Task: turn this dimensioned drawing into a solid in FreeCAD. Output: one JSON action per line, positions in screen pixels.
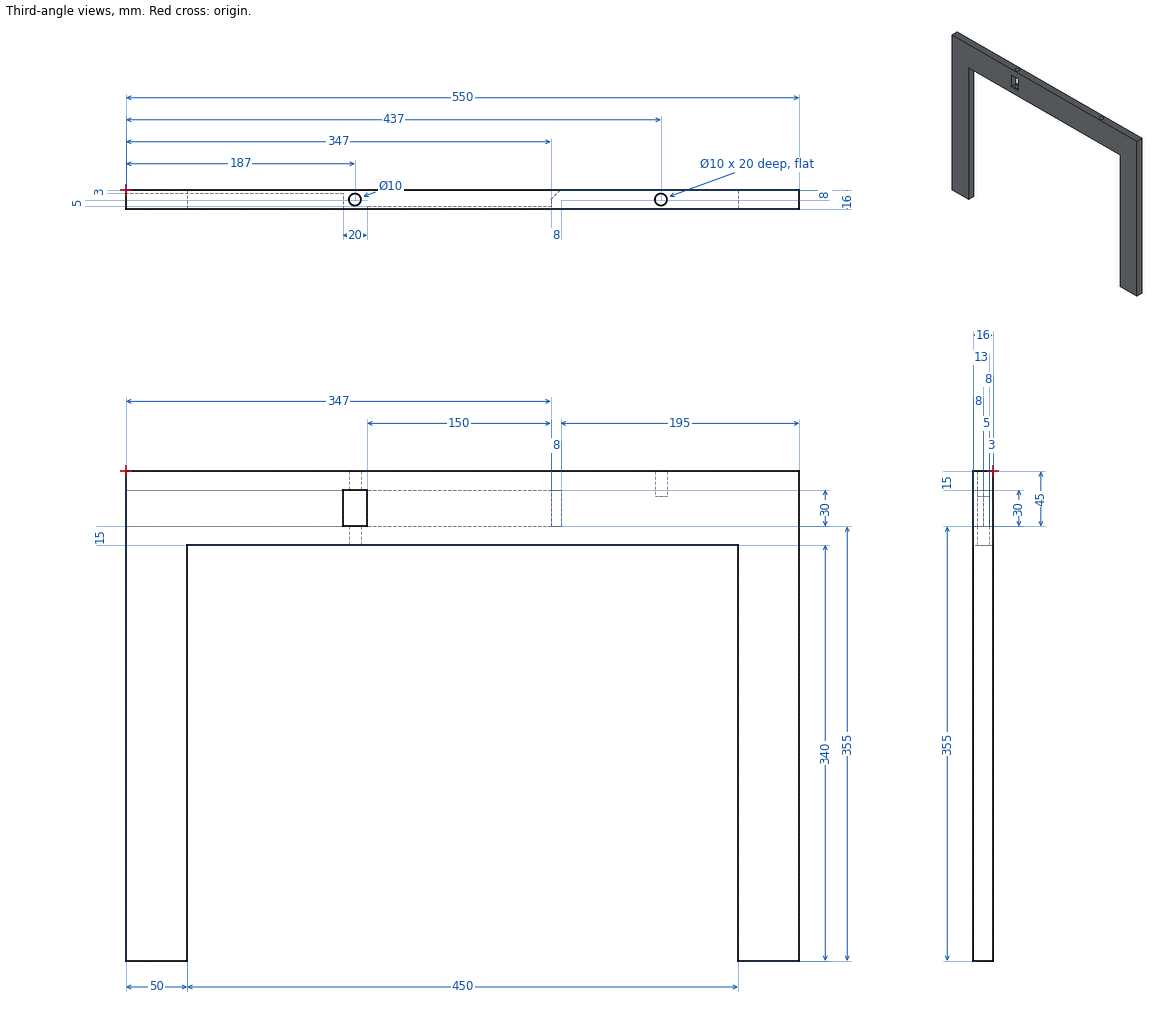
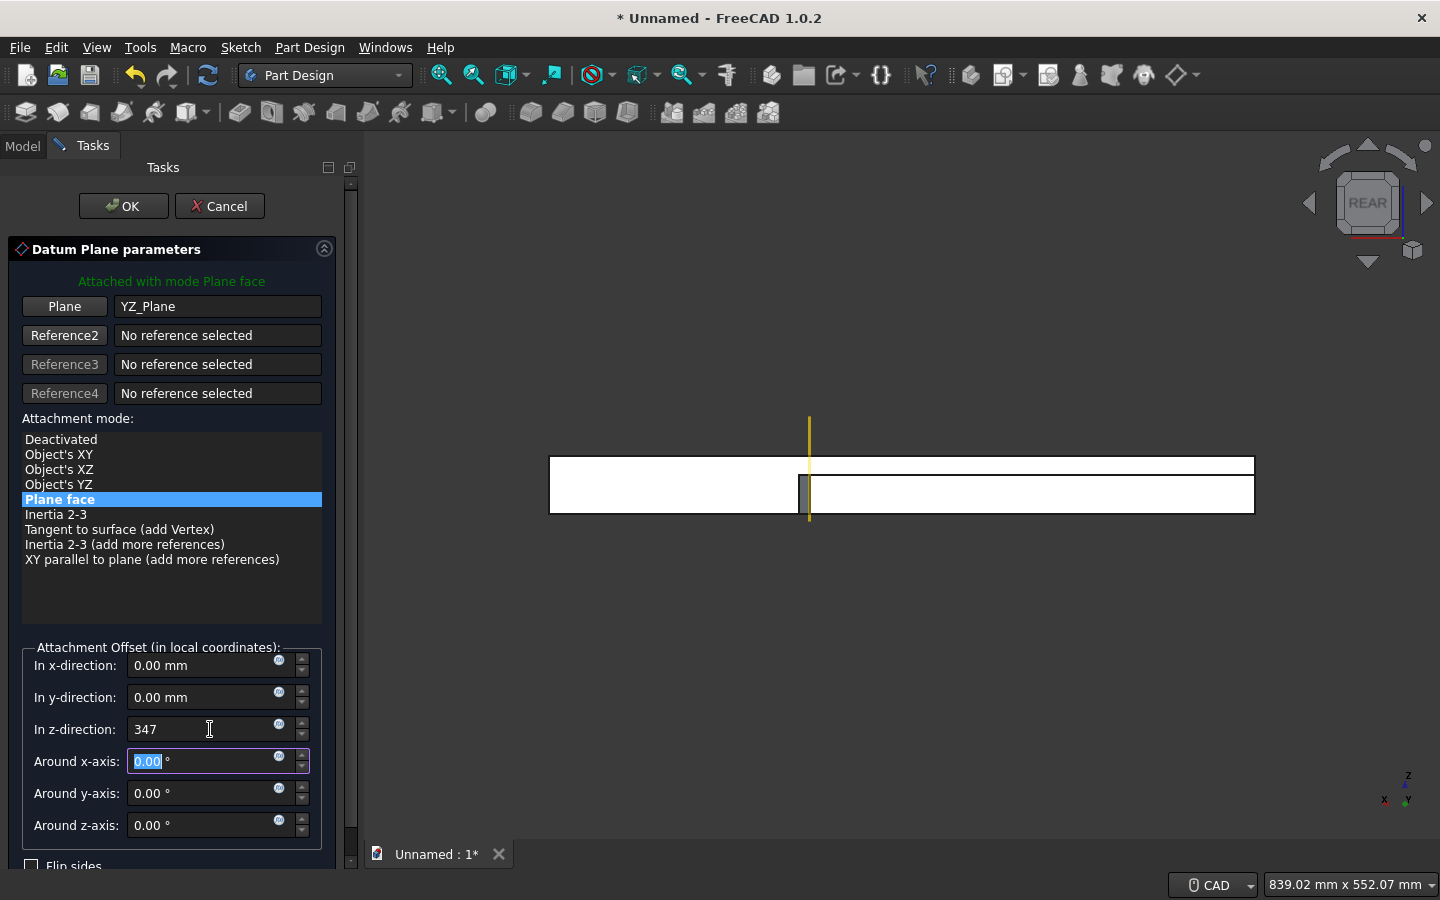
{"action": "left_click", "coordinate": [124, 206]}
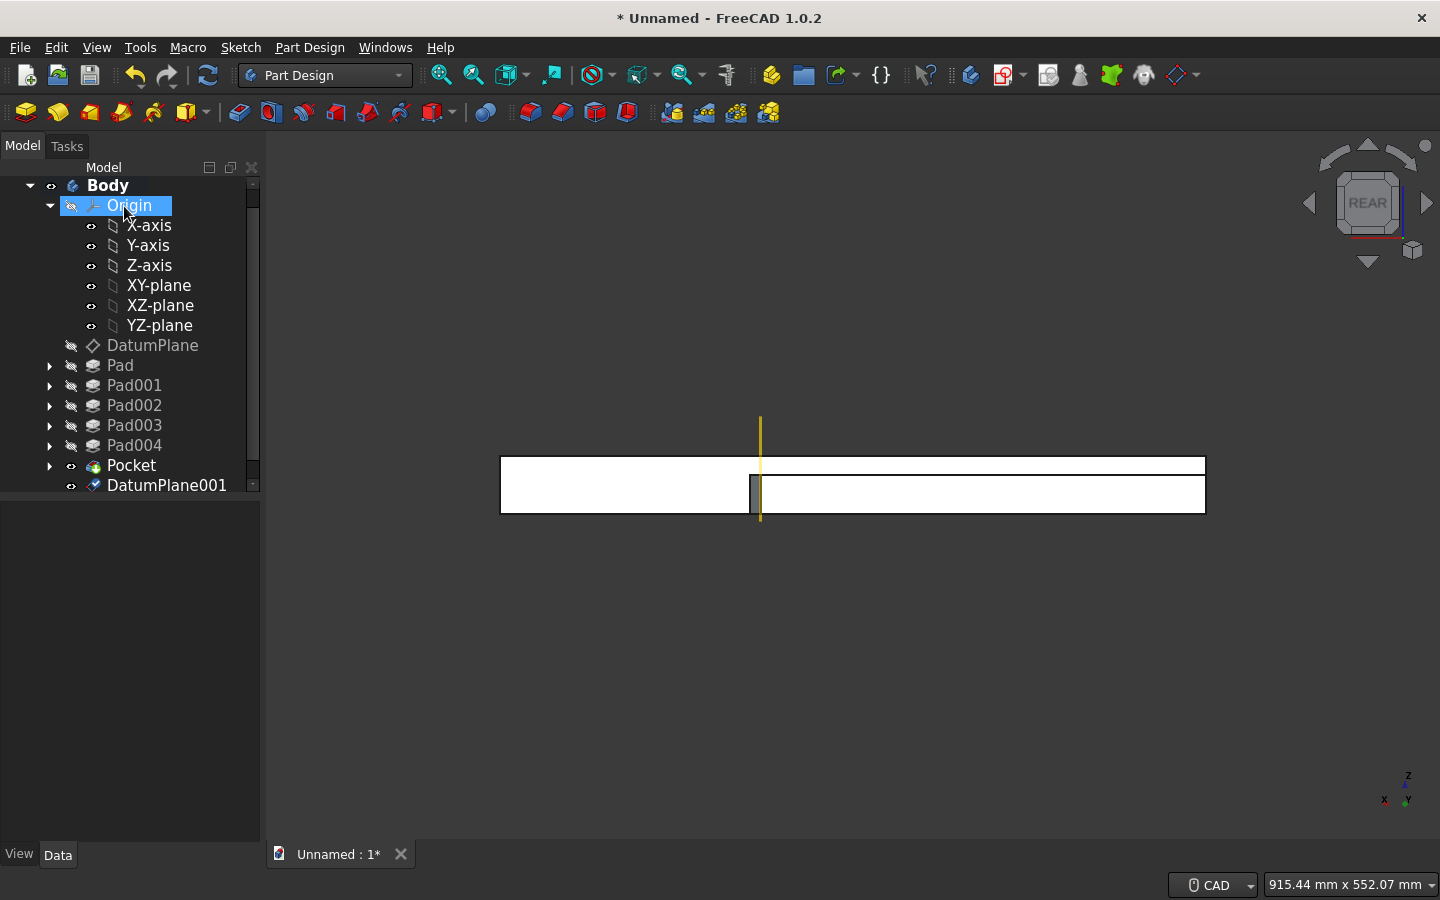
{"action": "left_click", "coordinate": [116, 486]}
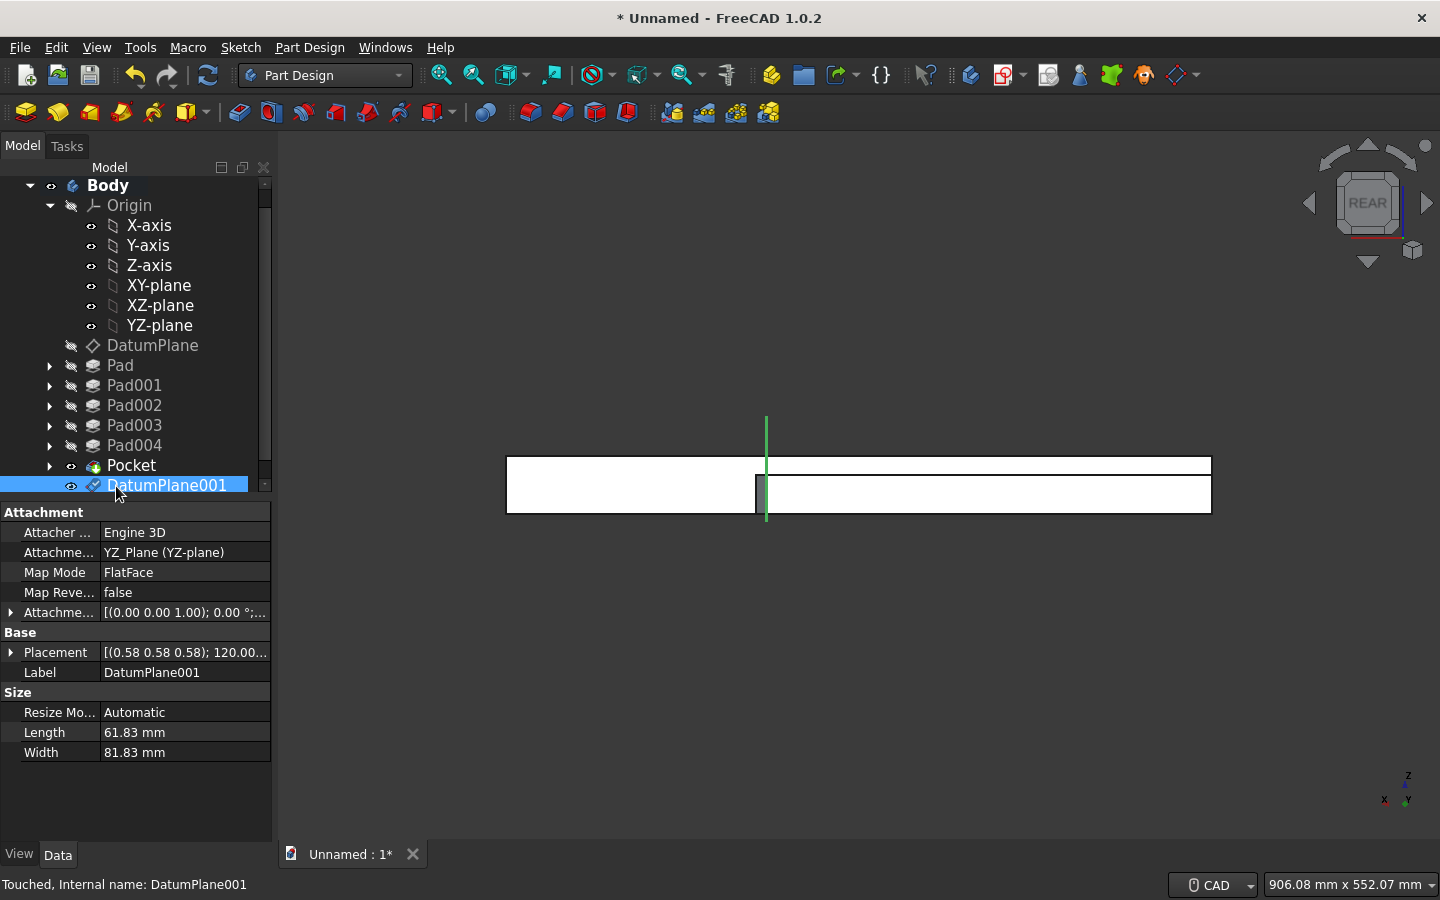
{"action": "left_click", "coordinate": [1004, 76]}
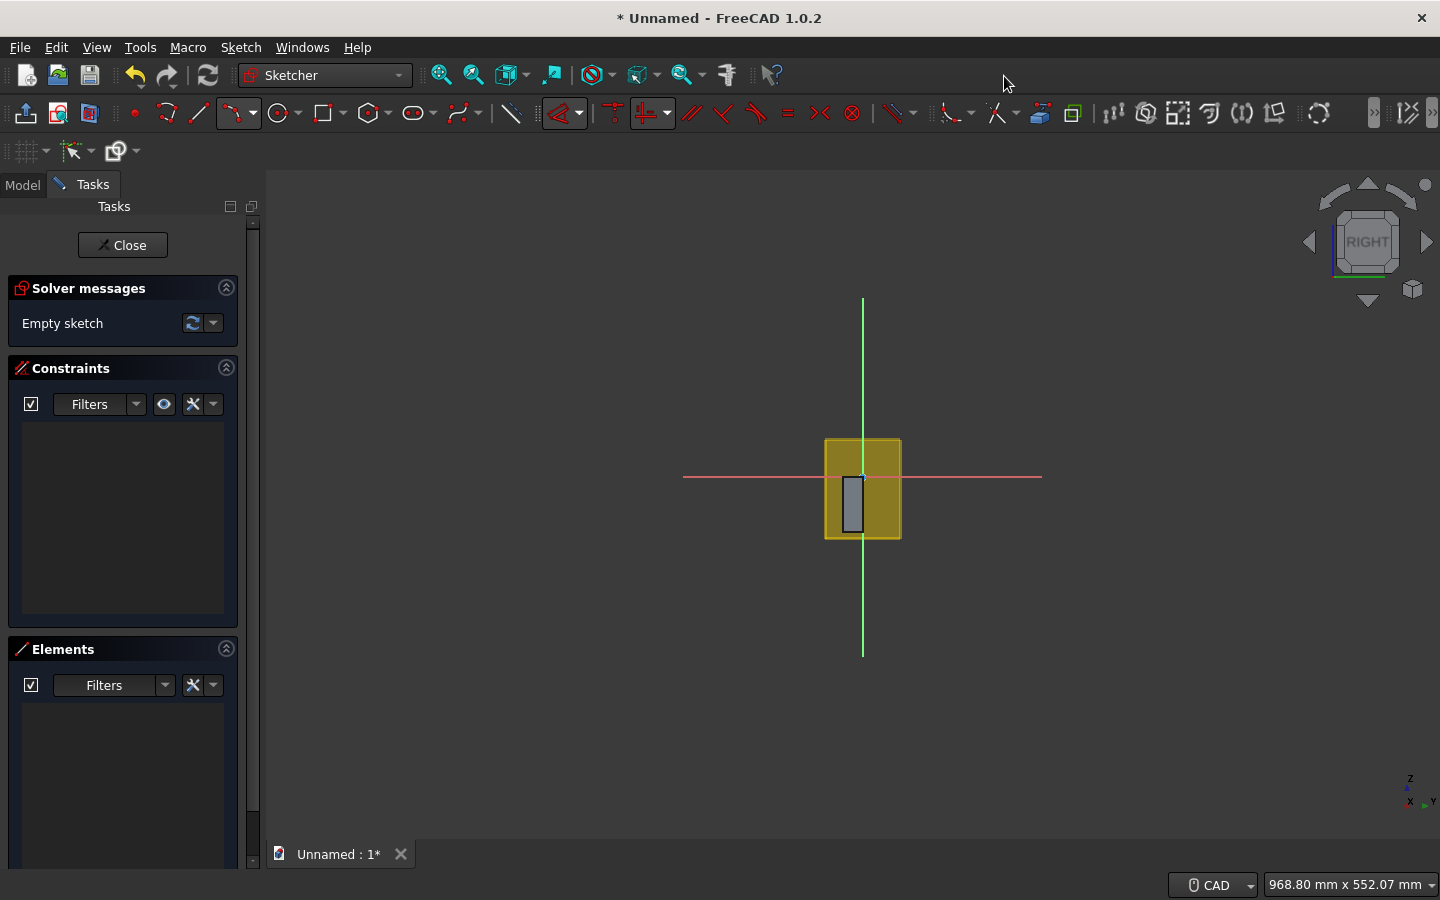
{"action": "left_click", "coordinate": [90, 114]}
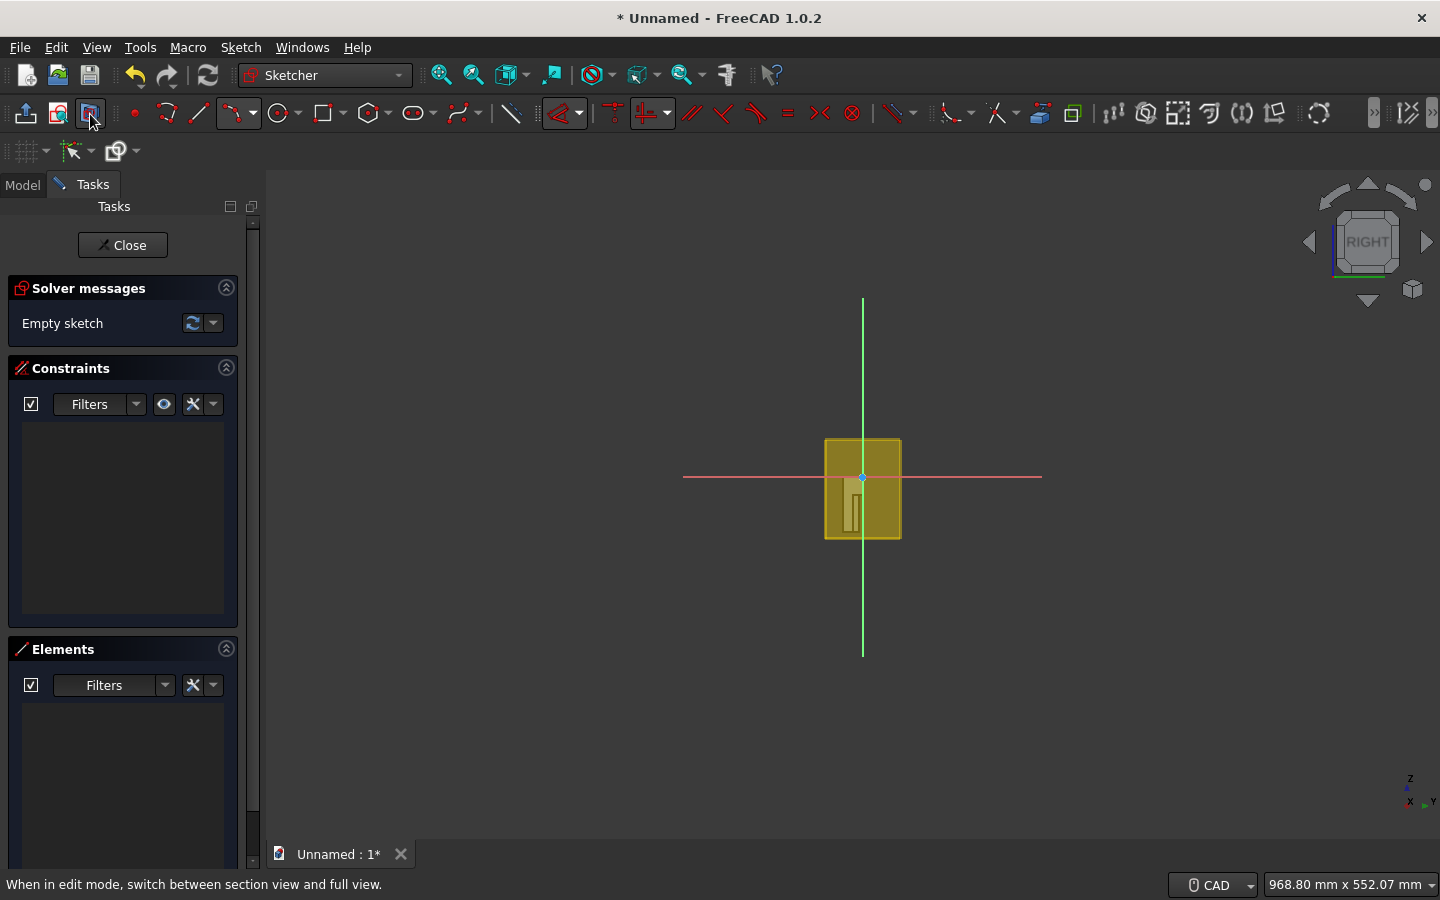
{"action": "scroll", "coordinate": [869, 505], "scroll_direction": "up", "scroll_amount": 10}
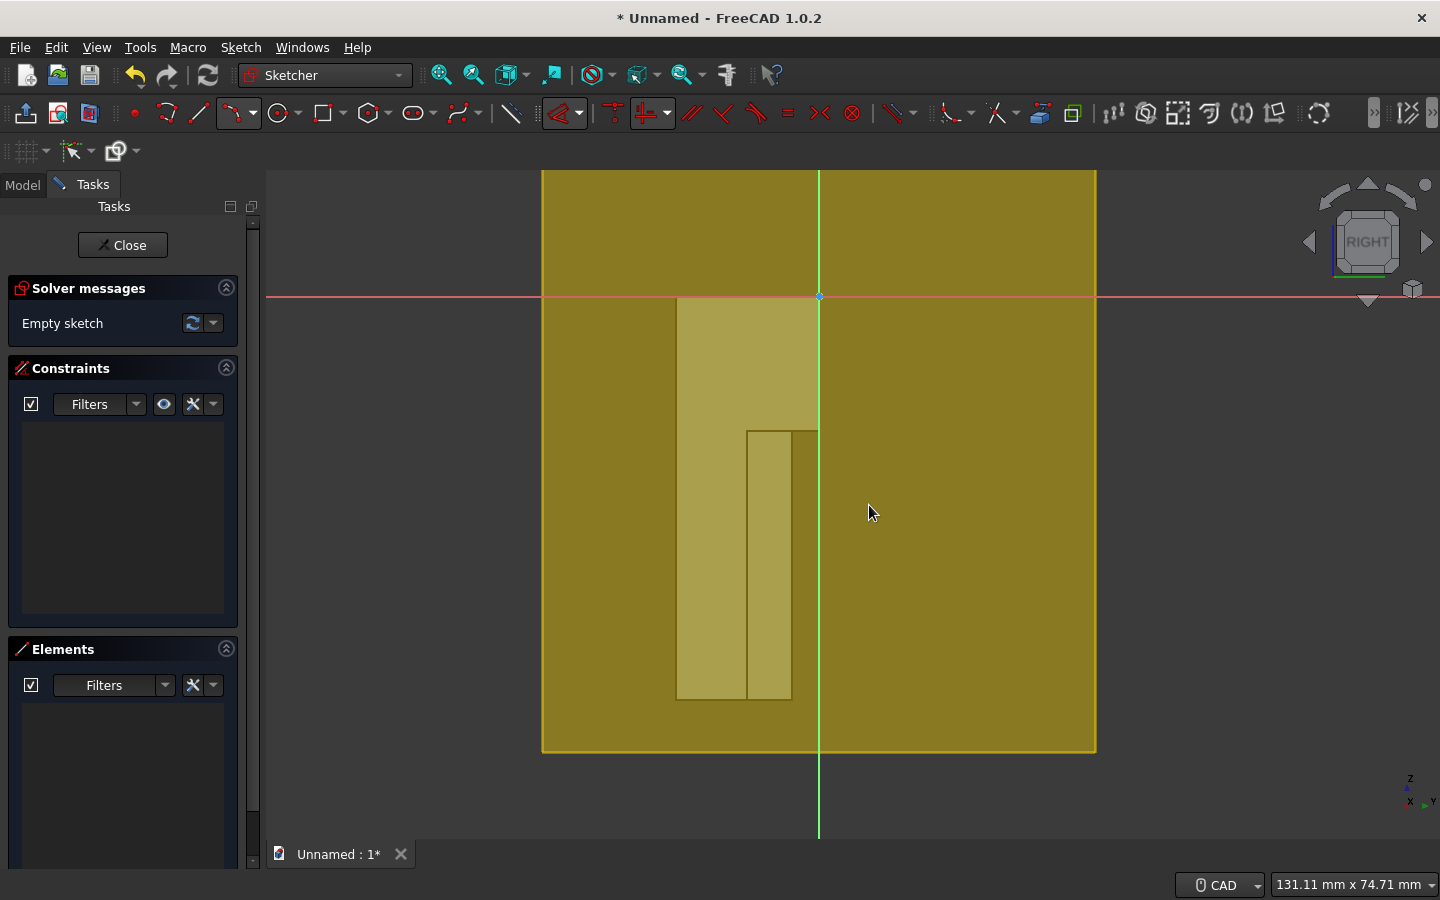
{"action": "left_click", "coordinate": [324, 114]}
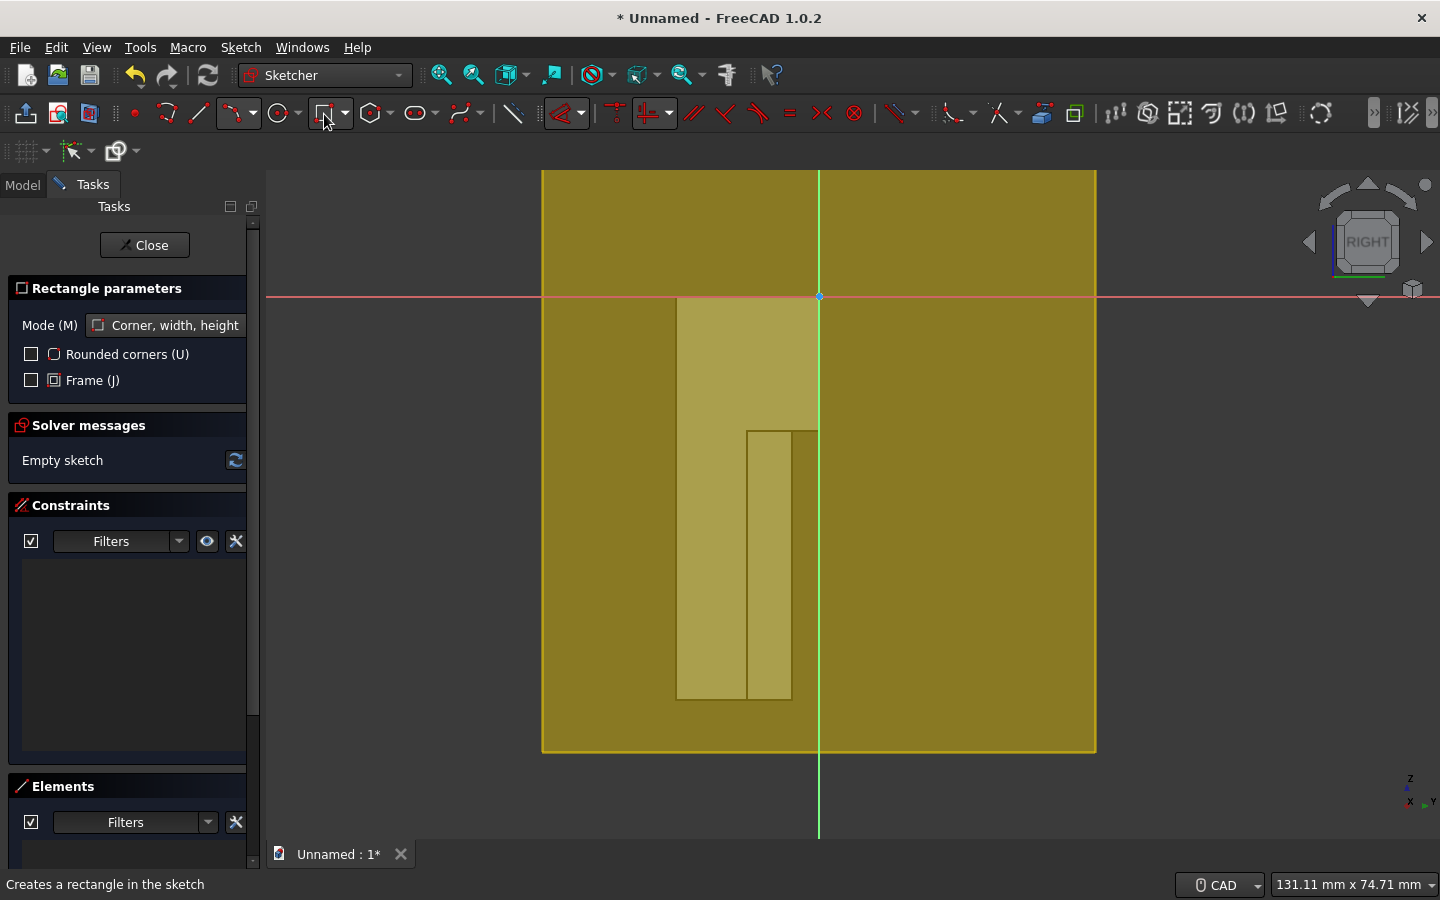
{"action": "left_click", "coordinate": [747, 431]}
{"action": "left_click", "coordinate": [792, 700]}
{"action": "key", "text": "Escape"}